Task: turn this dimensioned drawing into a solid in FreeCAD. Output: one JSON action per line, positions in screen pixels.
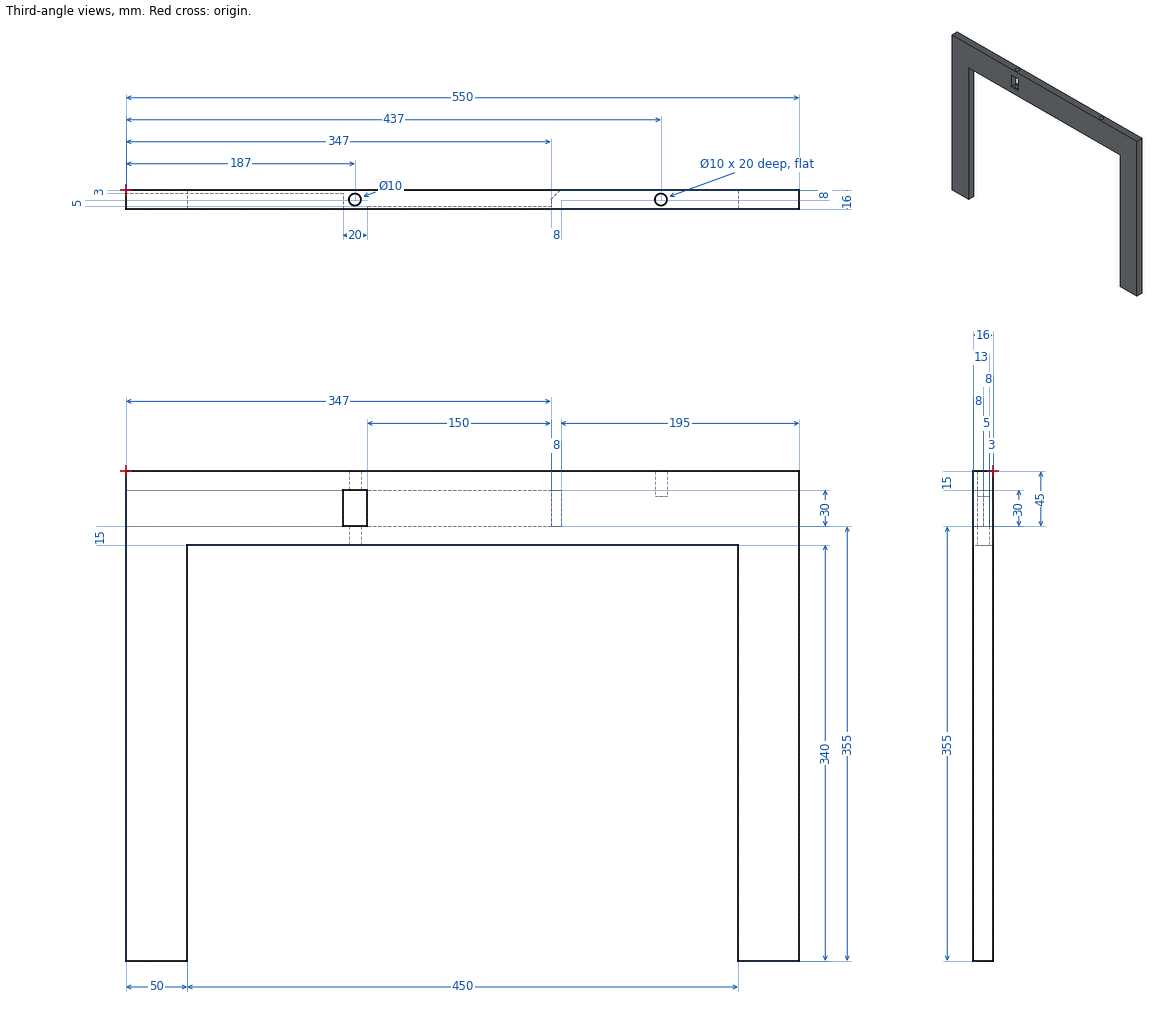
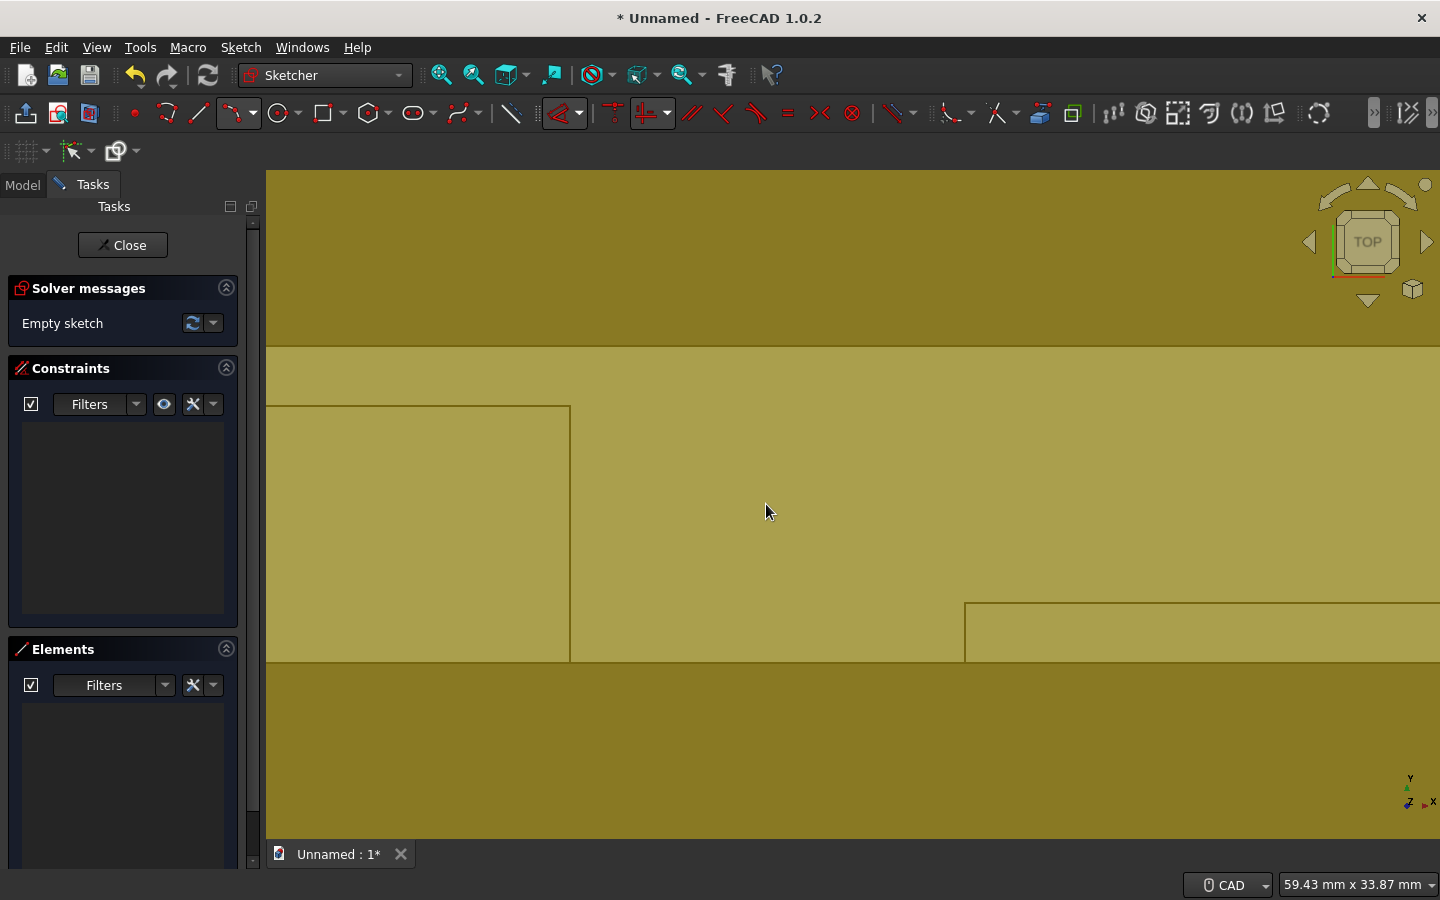
{"action": "scroll", "coordinate": [753, 504], "scroll_direction": "up", "scroll_amount": 4}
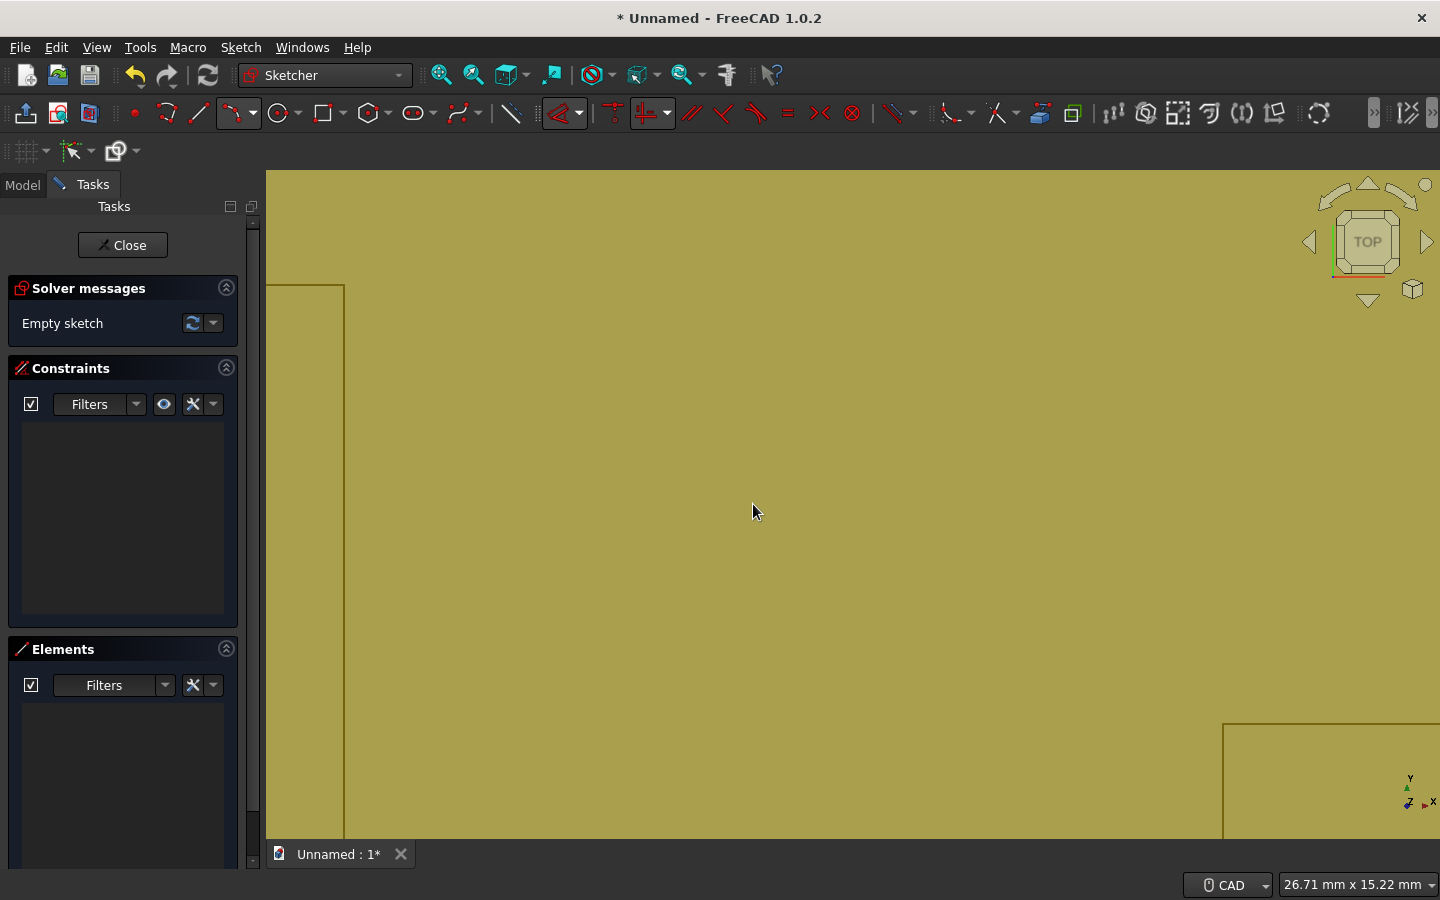
{"action": "left_click", "coordinate": [278, 114]}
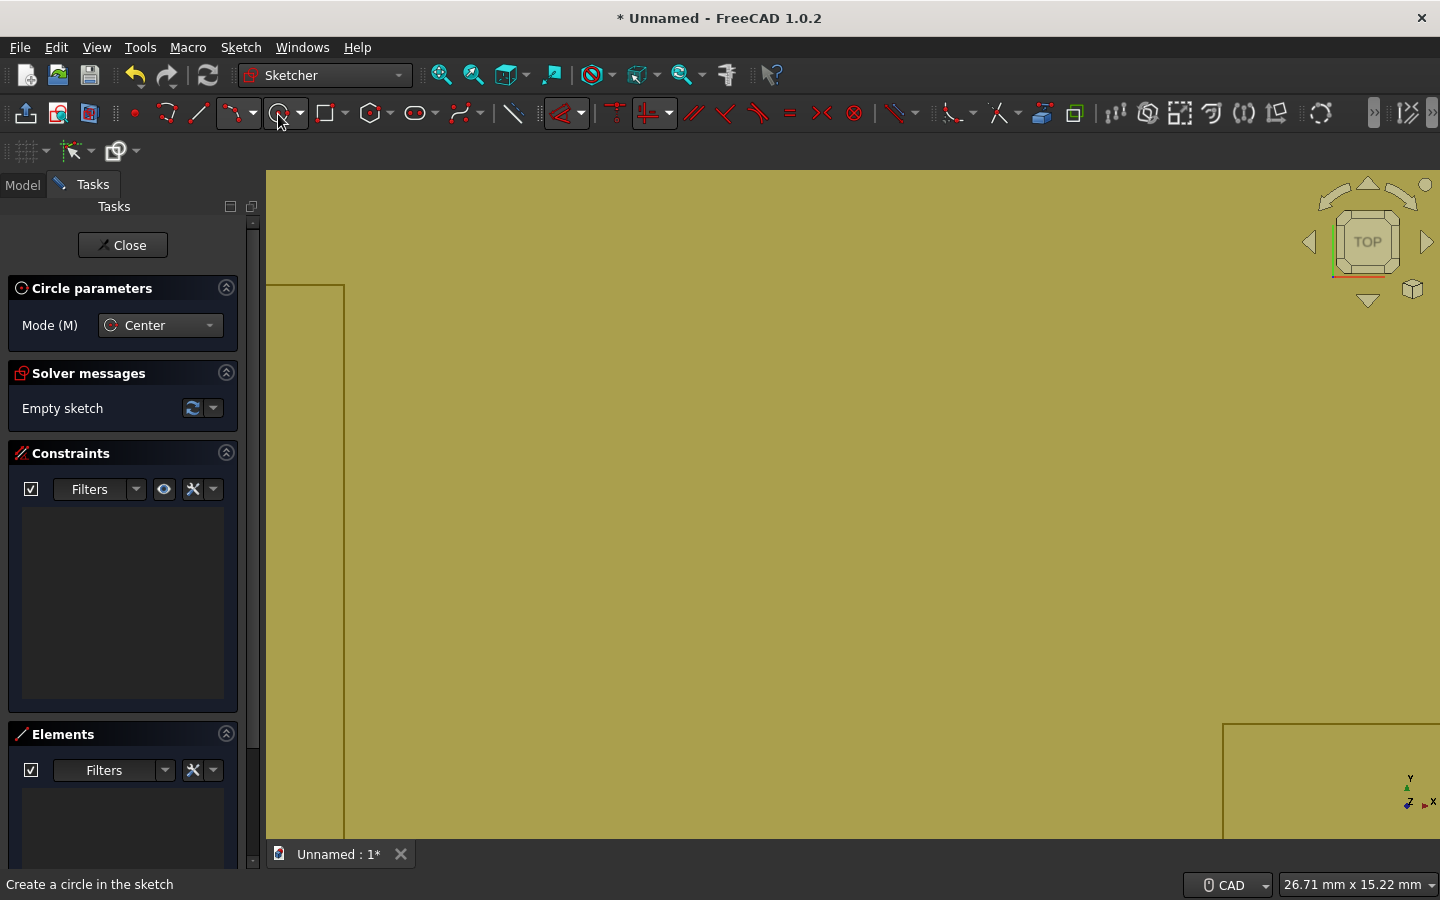
{"action": "left_click", "coordinate": [784, 504]}
{"action": "left_click", "coordinate": [939, 349]}
{"action": "key", "text": "Escape"}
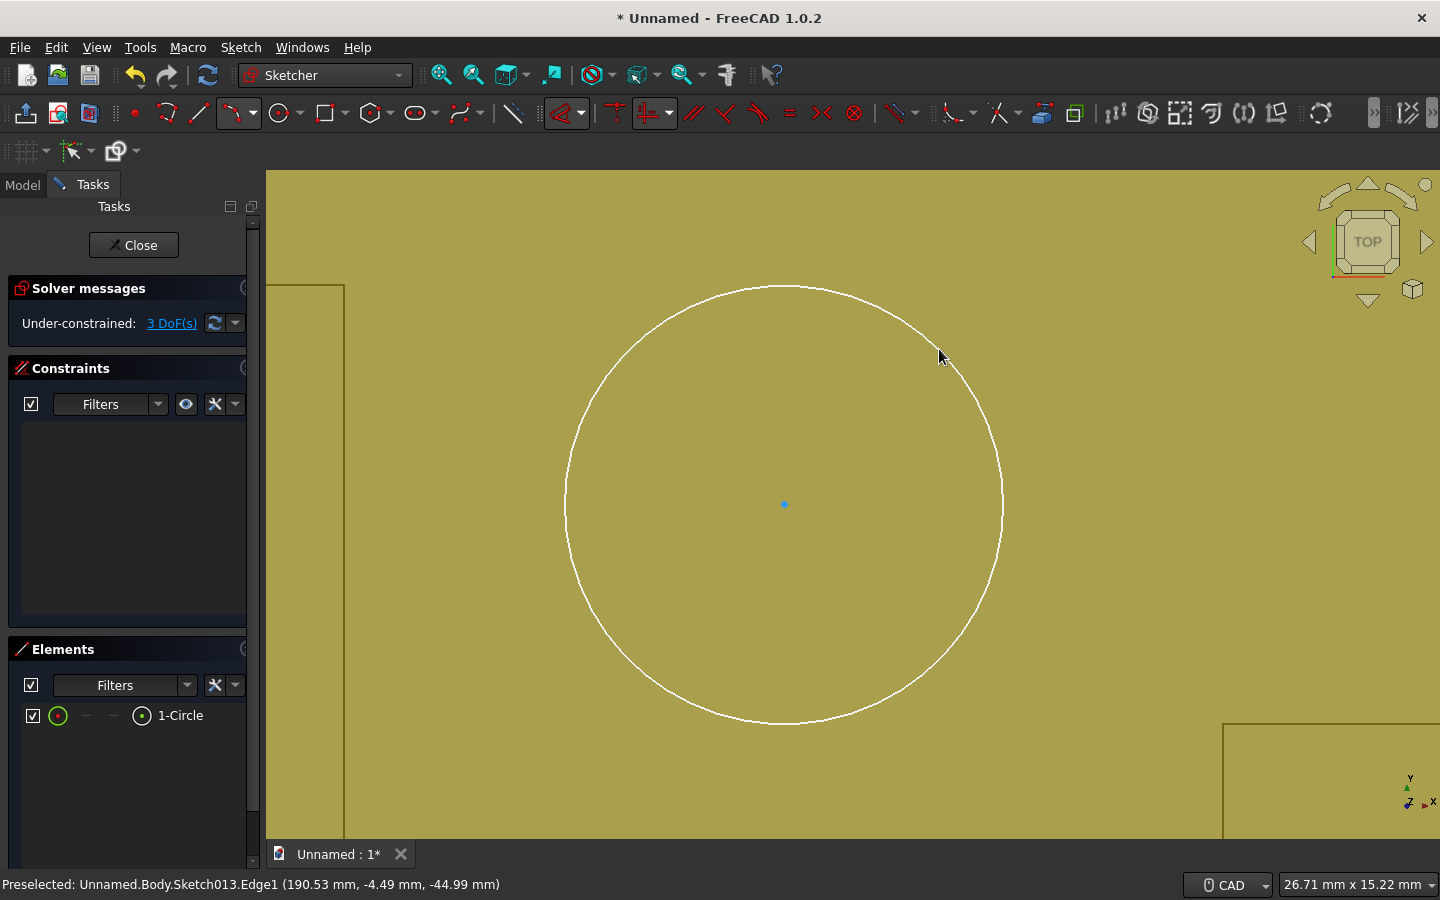
{"action": "left_click", "coordinate": [939, 350]}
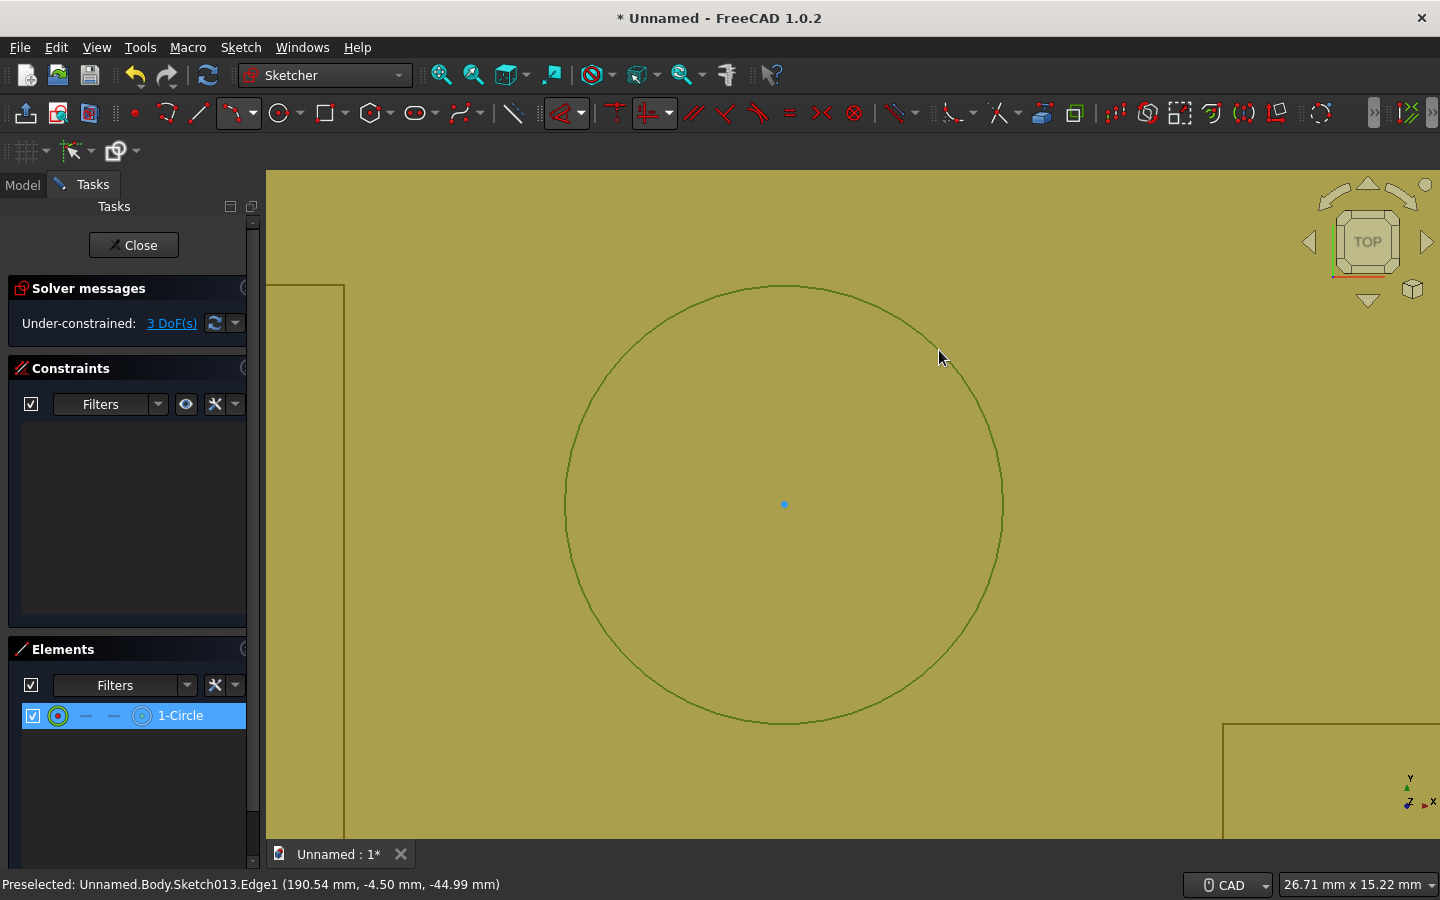
{"action": "left_click", "coordinate": [584, 114]}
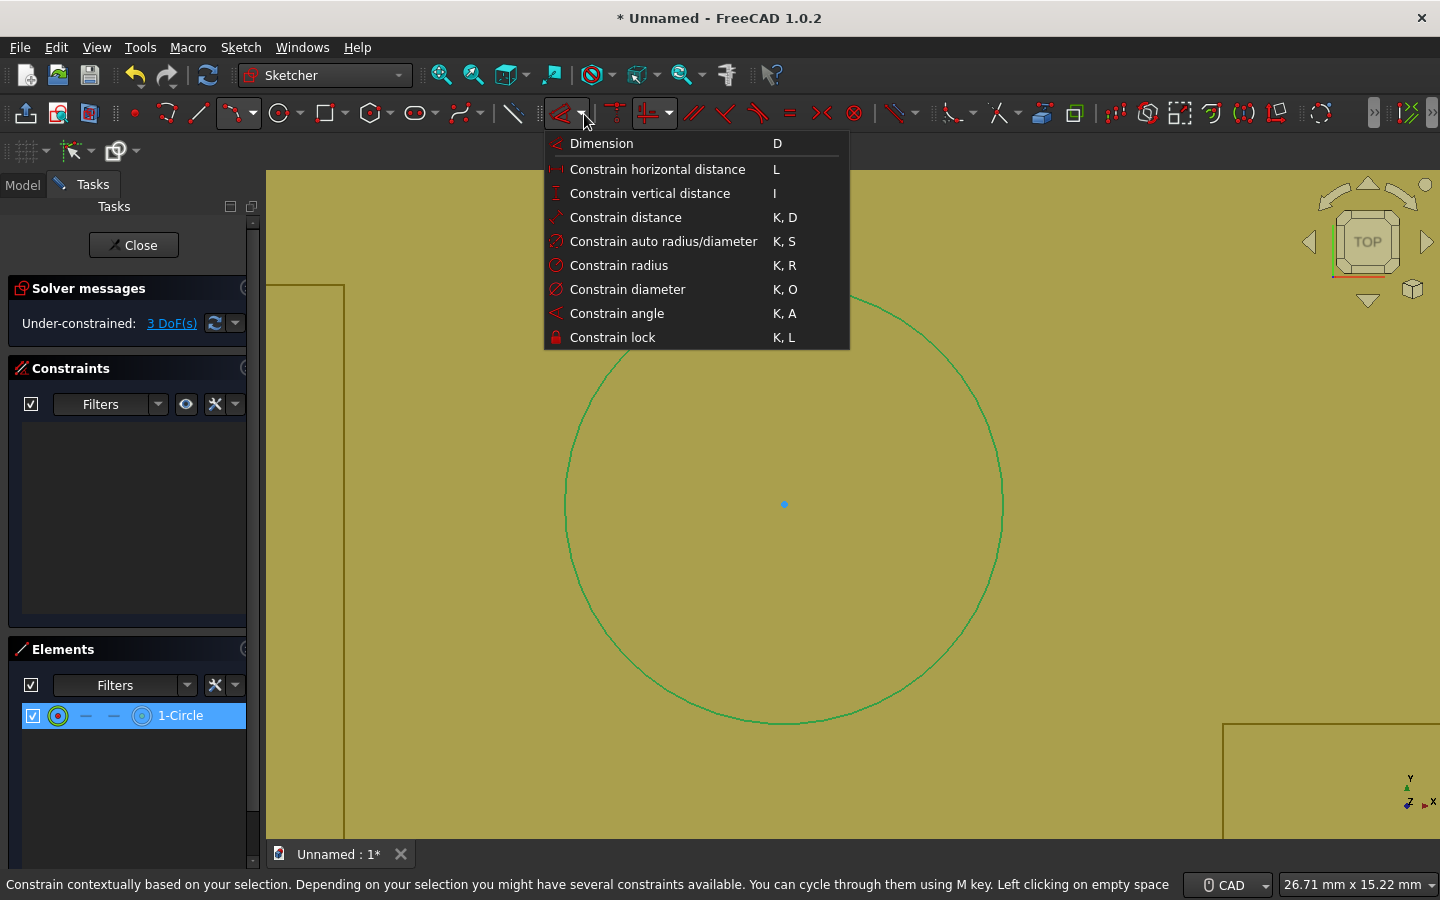
{"action": "left_click", "coordinate": [697, 289]}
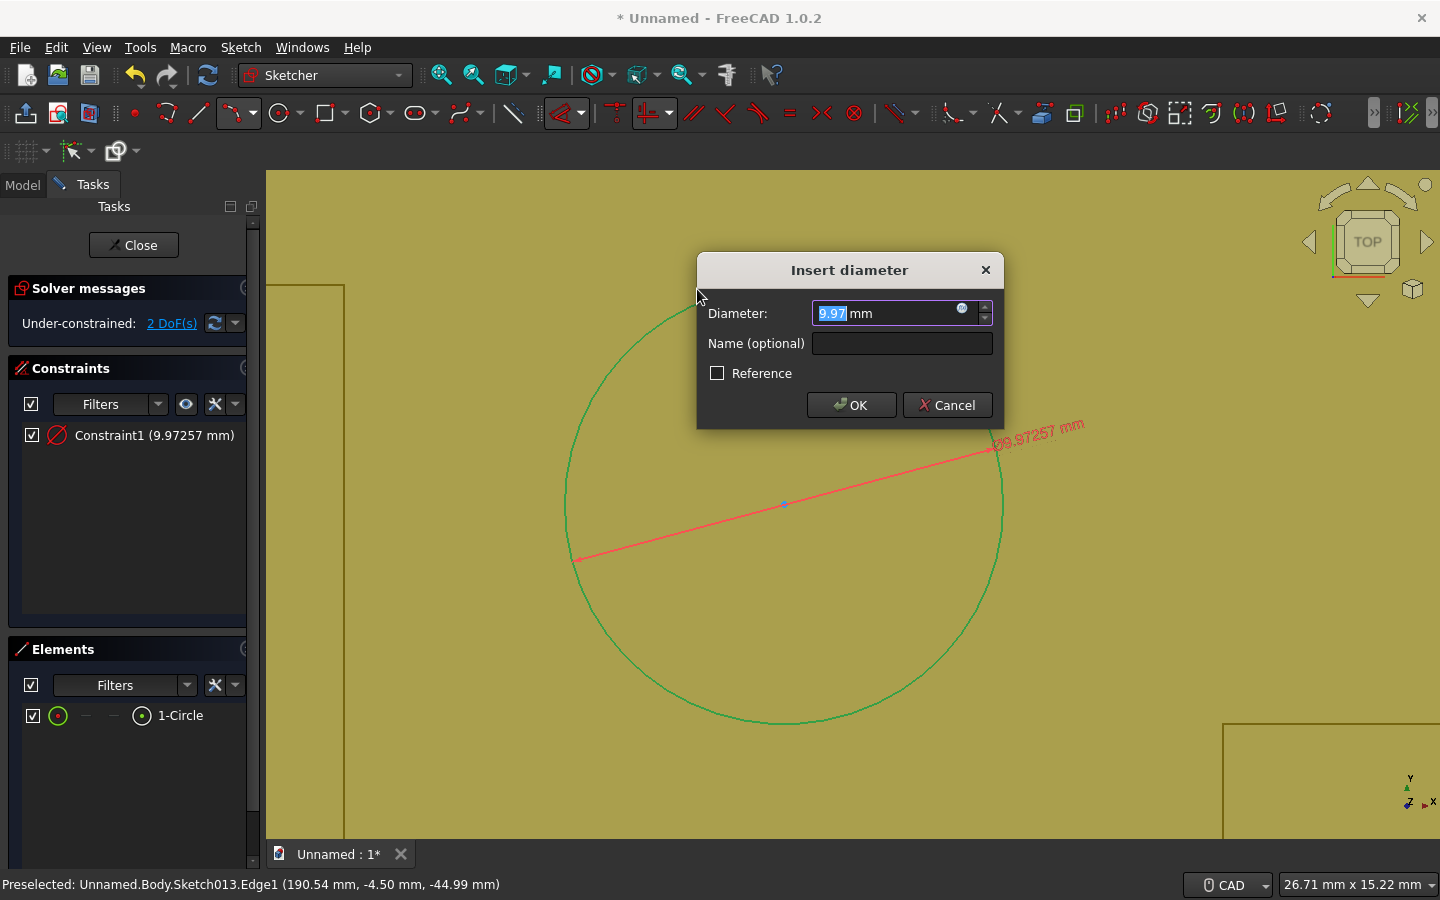
{"action": "type", "text": "10"}
{"action": "key", "text": "Return"}